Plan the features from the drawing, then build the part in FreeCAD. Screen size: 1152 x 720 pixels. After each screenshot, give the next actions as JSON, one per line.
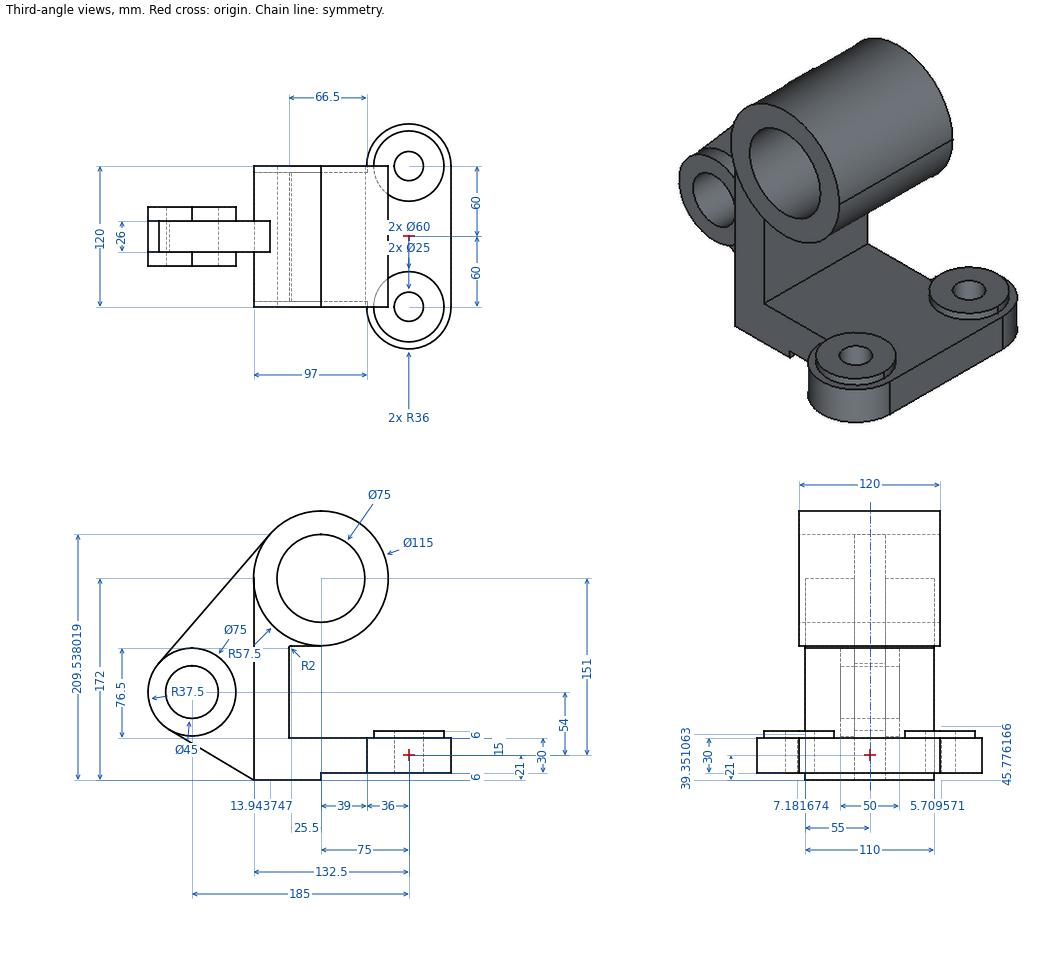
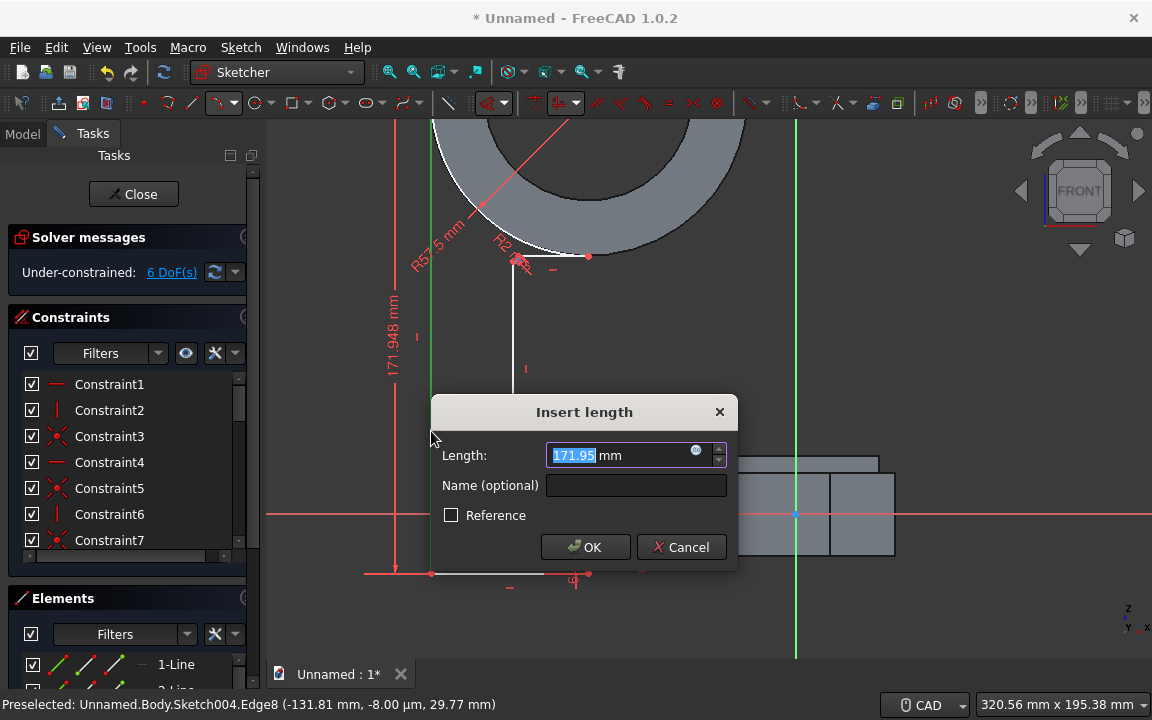
{"action": "type", "text": "172"}
{"action": "key", "text": "Return"}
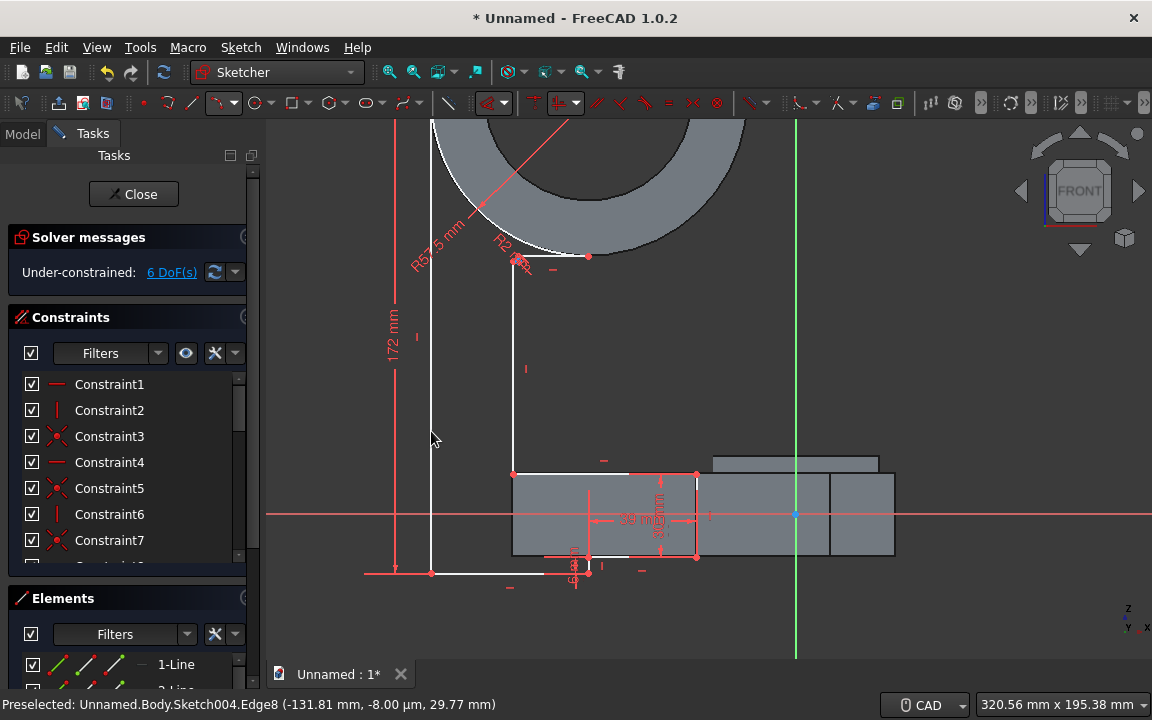
{"action": "left_click", "coordinate": [588, 256]}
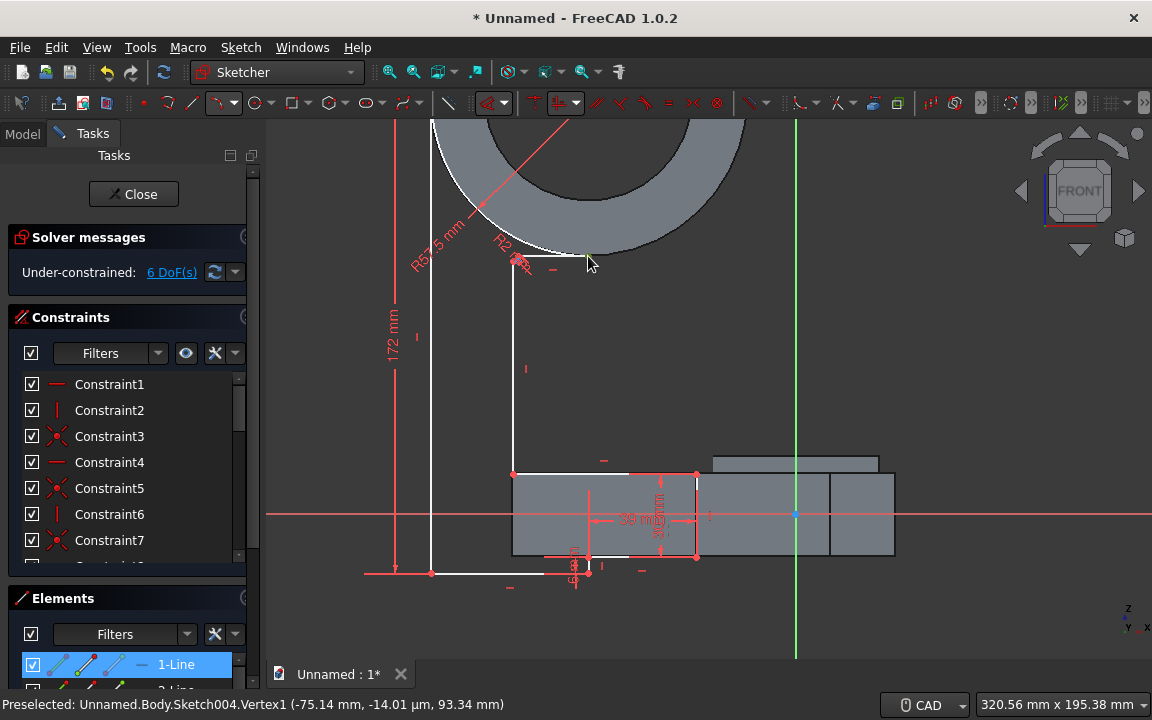
{"action": "key", "text": "l"}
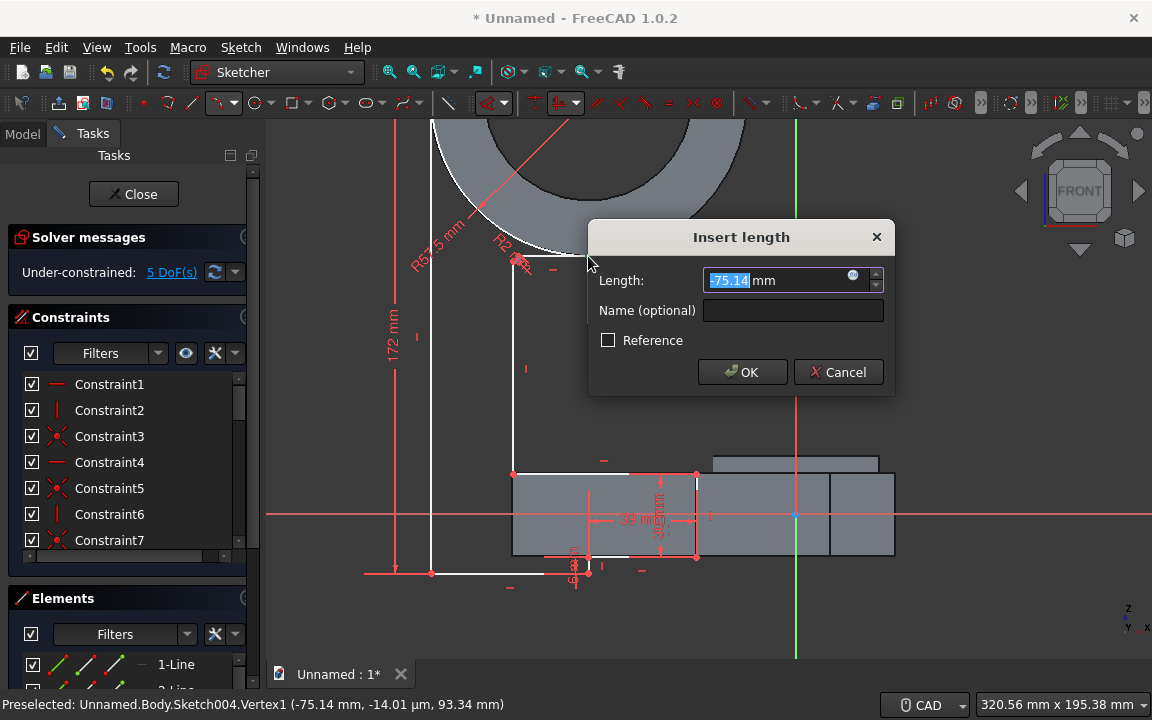
{"action": "type", "text": "-75"}
{"action": "key", "text": "Return"}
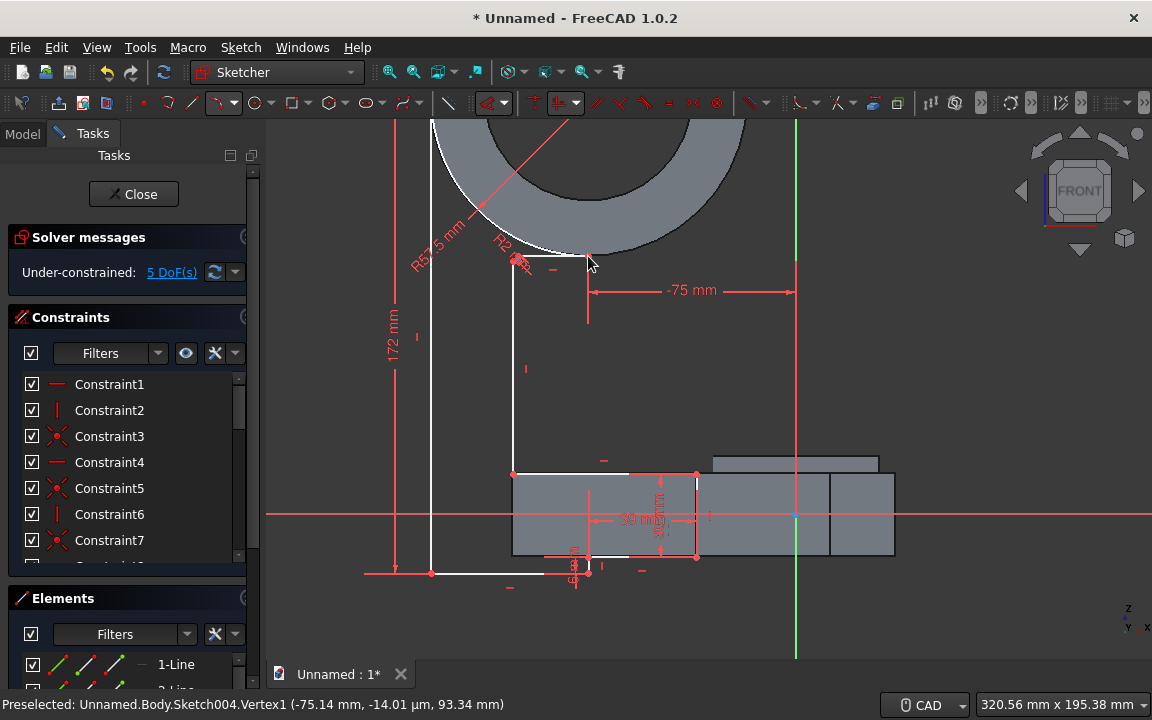
{"action": "left_click", "coordinate": [513, 474]}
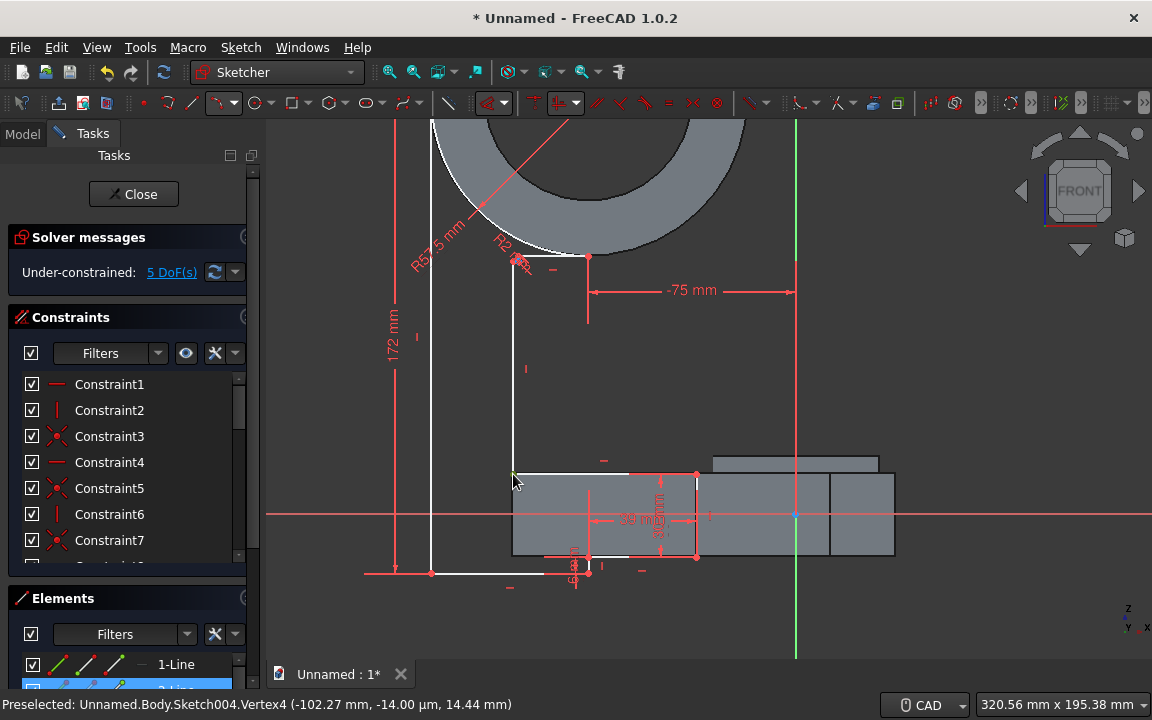
{"action": "key", "text": "i"}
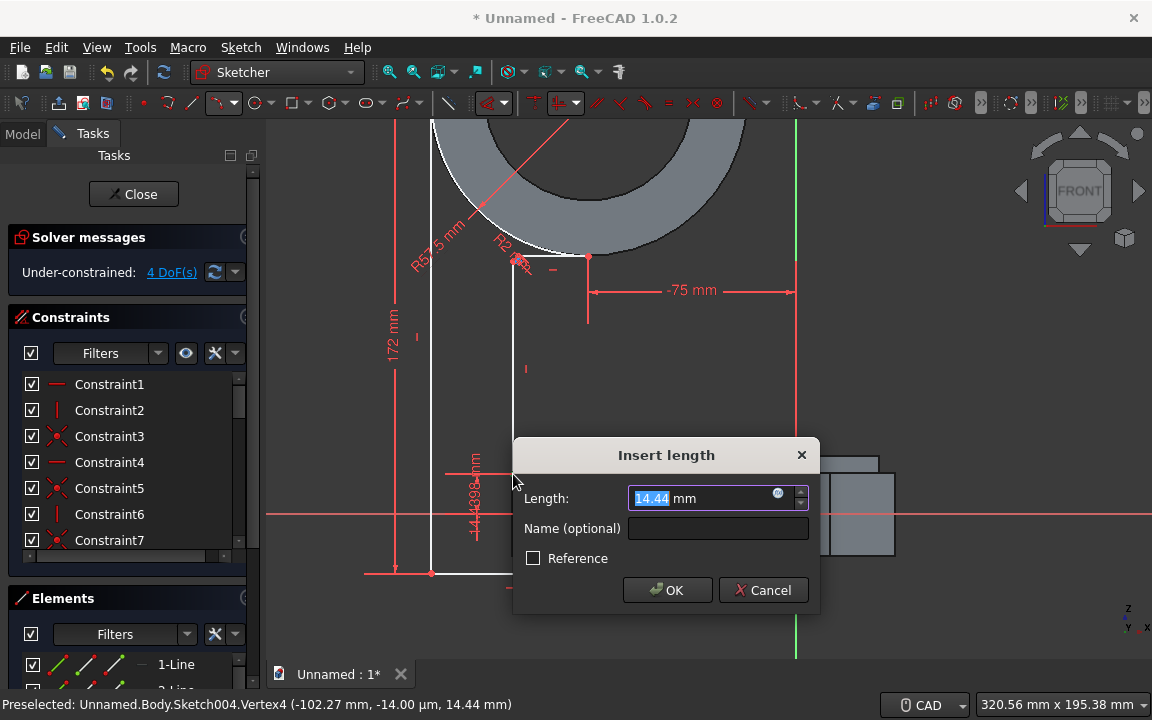
{"action": "type", "text": "15"}
{"action": "key", "text": "Return"}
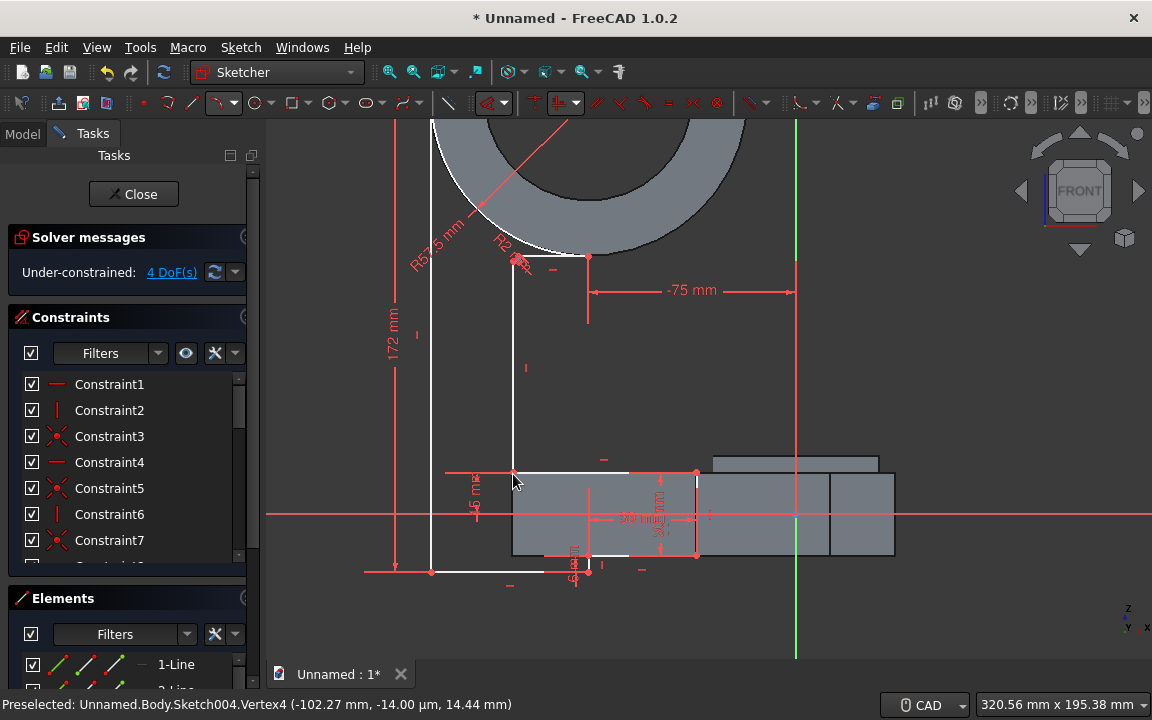
{"action": "left_click", "coordinate": [697, 473]}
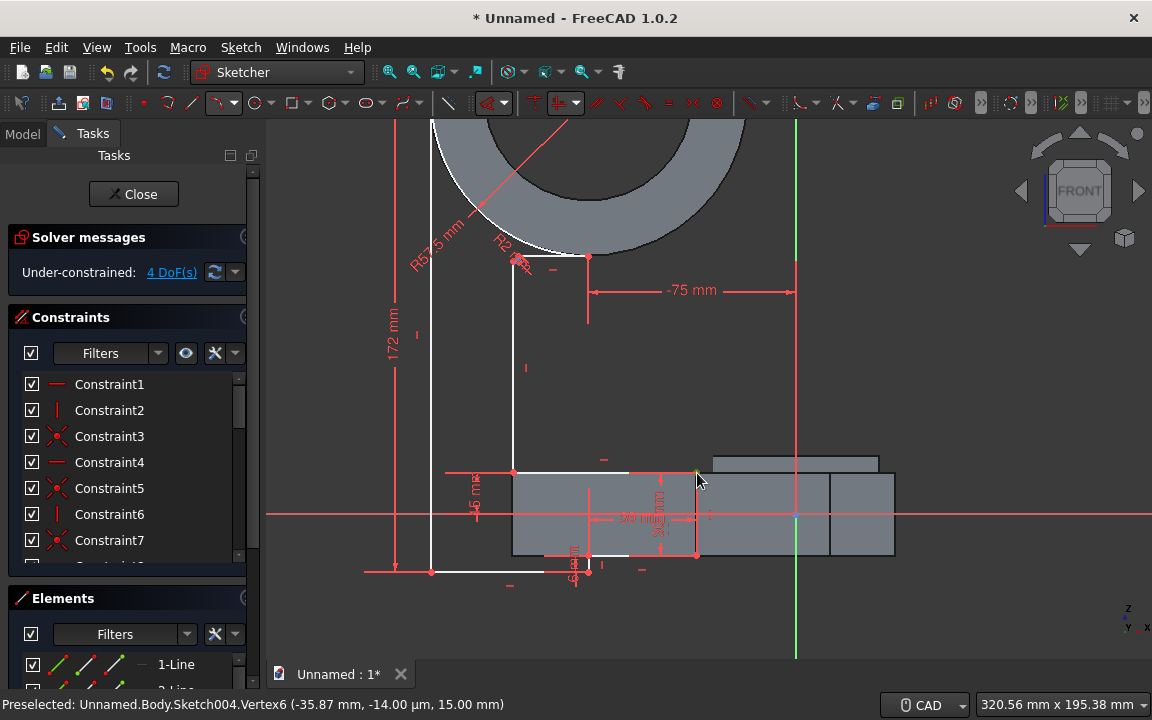
{"action": "key", "text": "l"}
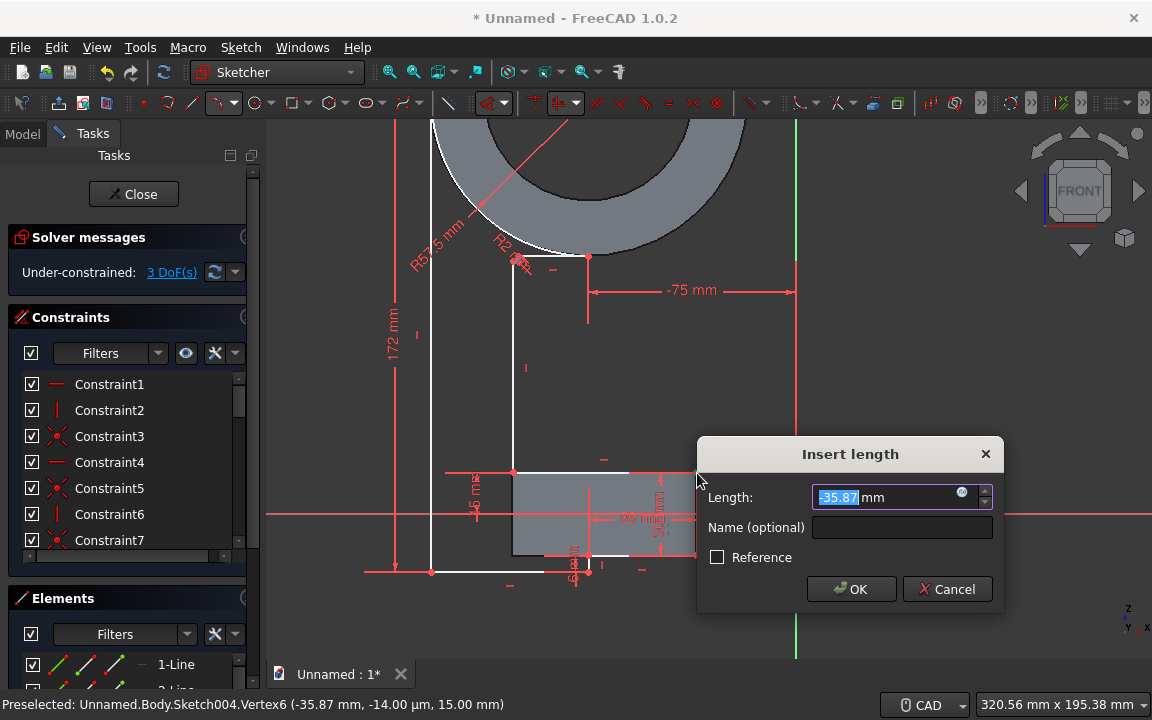
{"action": "type", "text": "-36"}
{"action": "key", "text": "Return"}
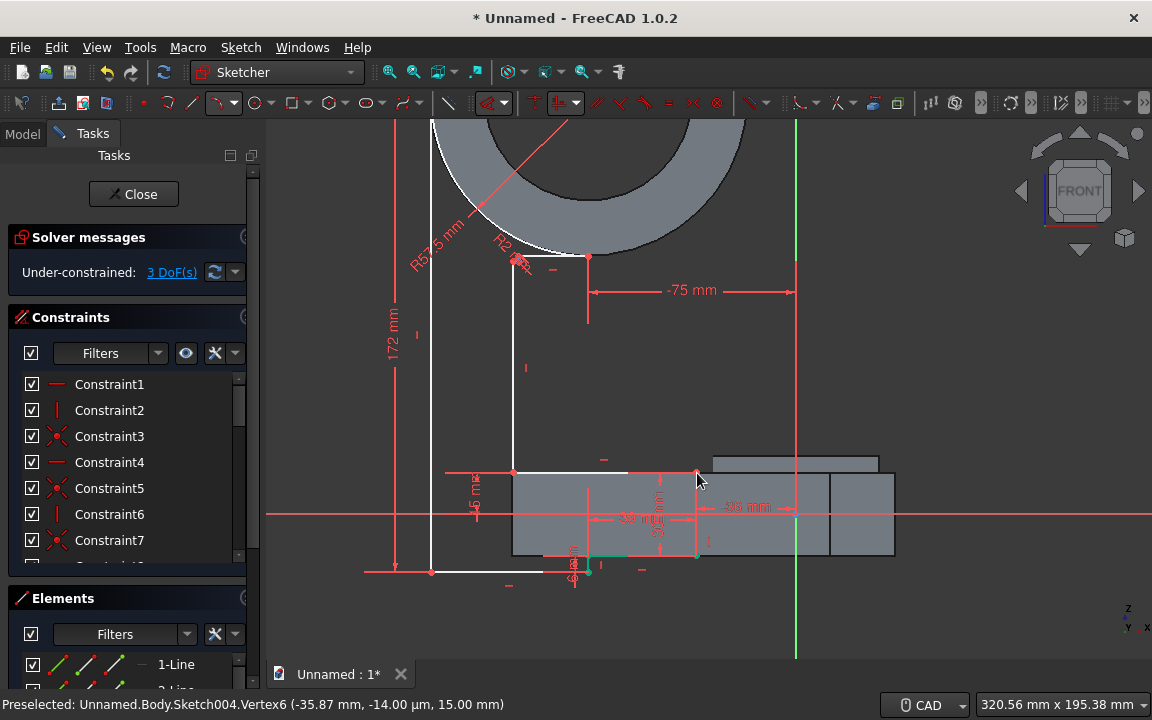
{"action": "scroll", "coordinate": [697, 500], "scroll_direction": "down", "scroll_amount": 2}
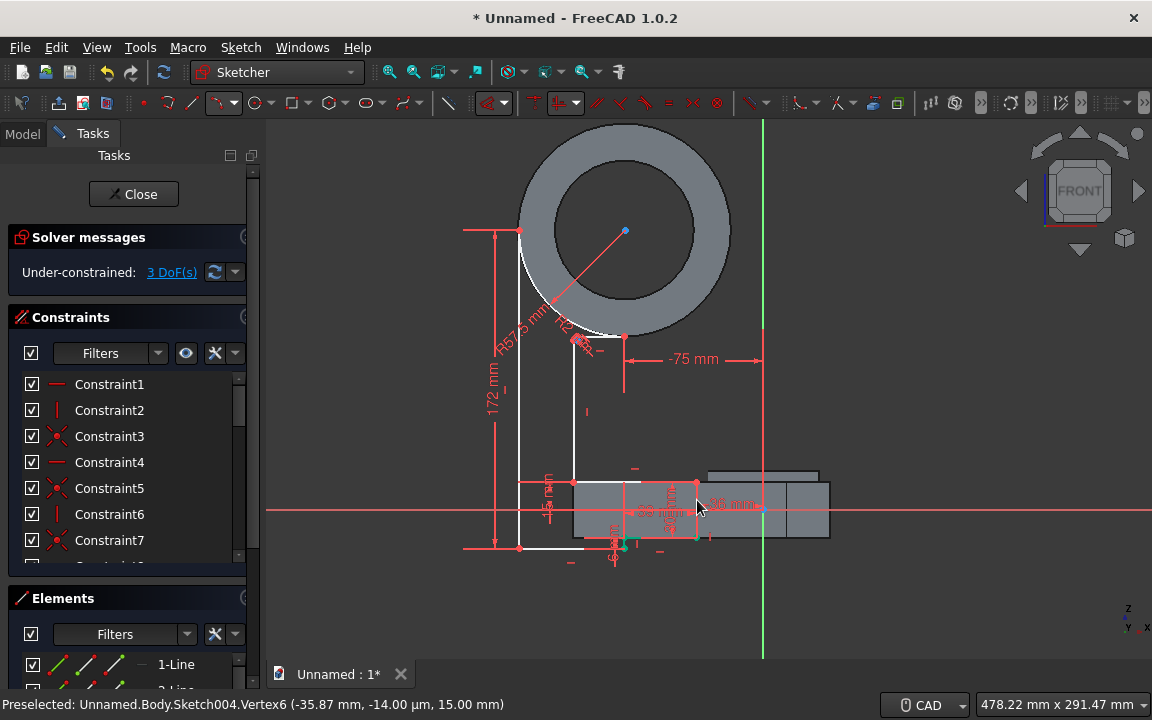
{"action": "left_click", "coordinate": [626, 230]}